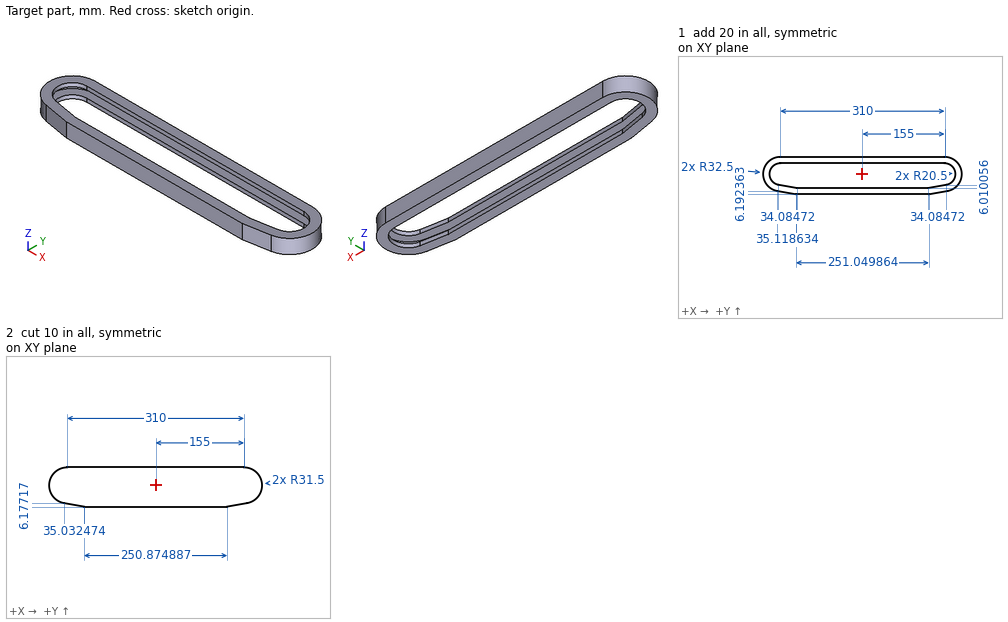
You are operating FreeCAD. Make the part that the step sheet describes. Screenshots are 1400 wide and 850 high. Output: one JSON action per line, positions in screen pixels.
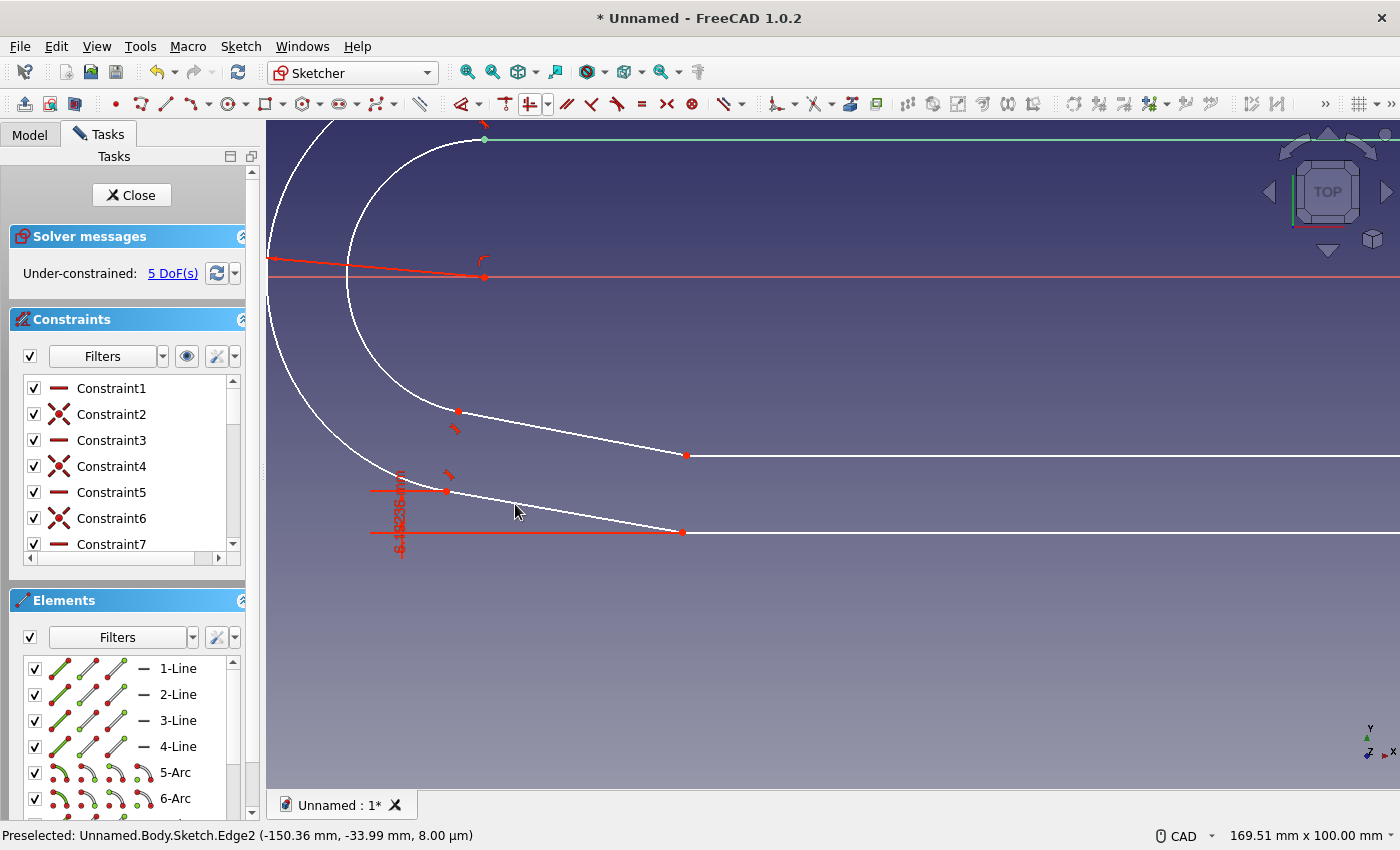
{"action": "scroll", "coordinate": [517, 506], "scroll_direction": "down", "scroll_amount": 7}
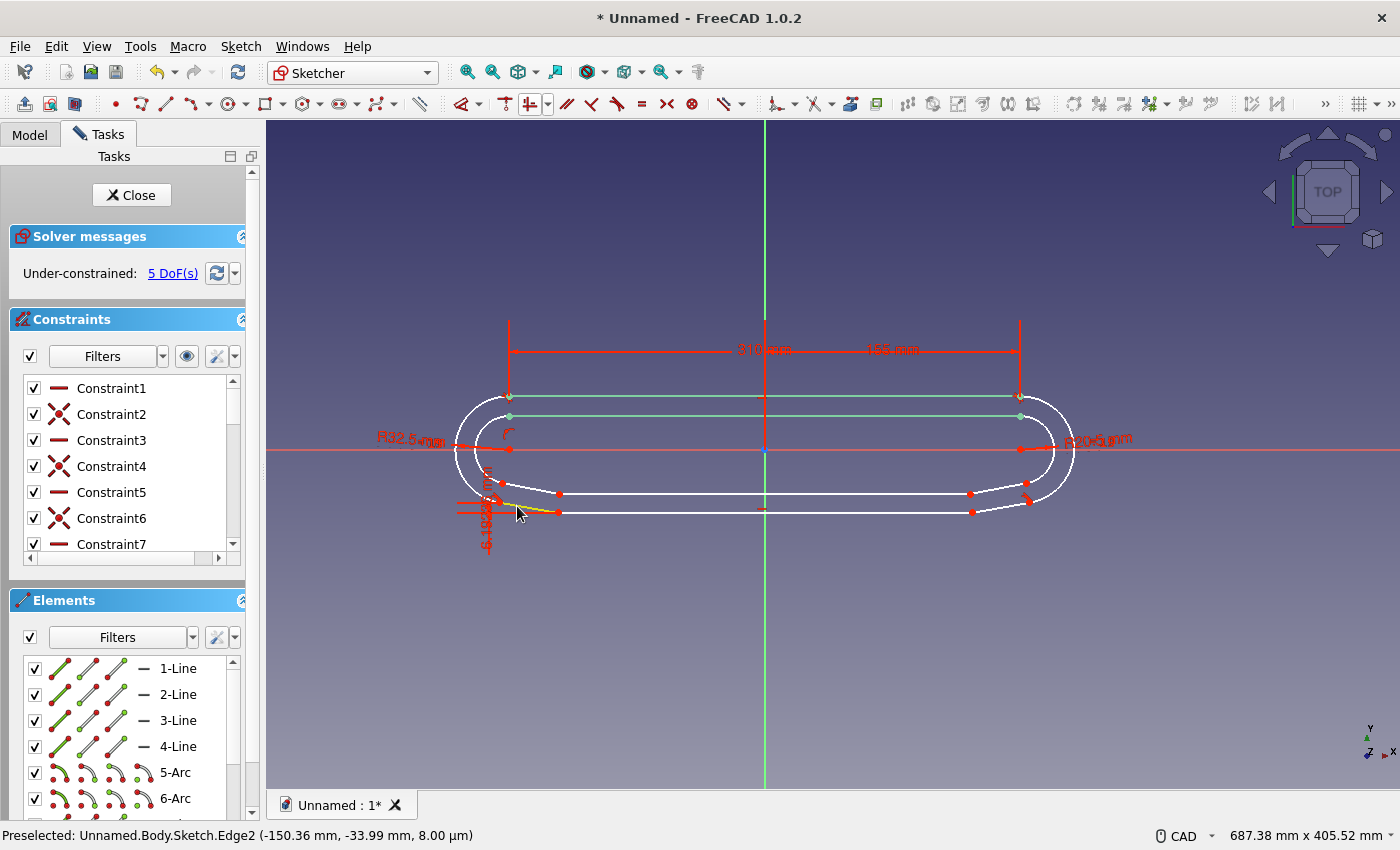
{"action": "left_click", "coordinate": [1010, 486]}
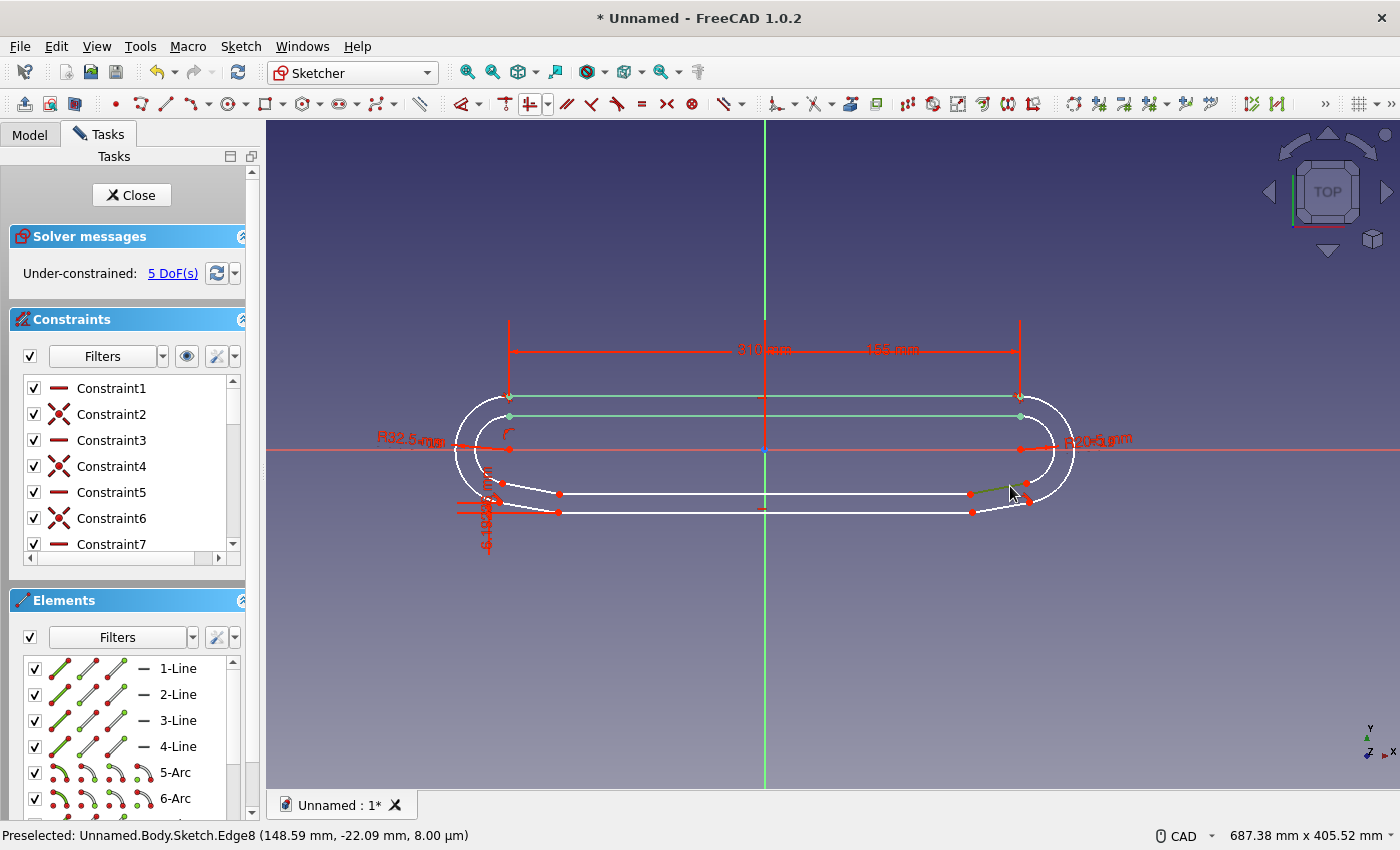
{"action": "key", "text": "l"}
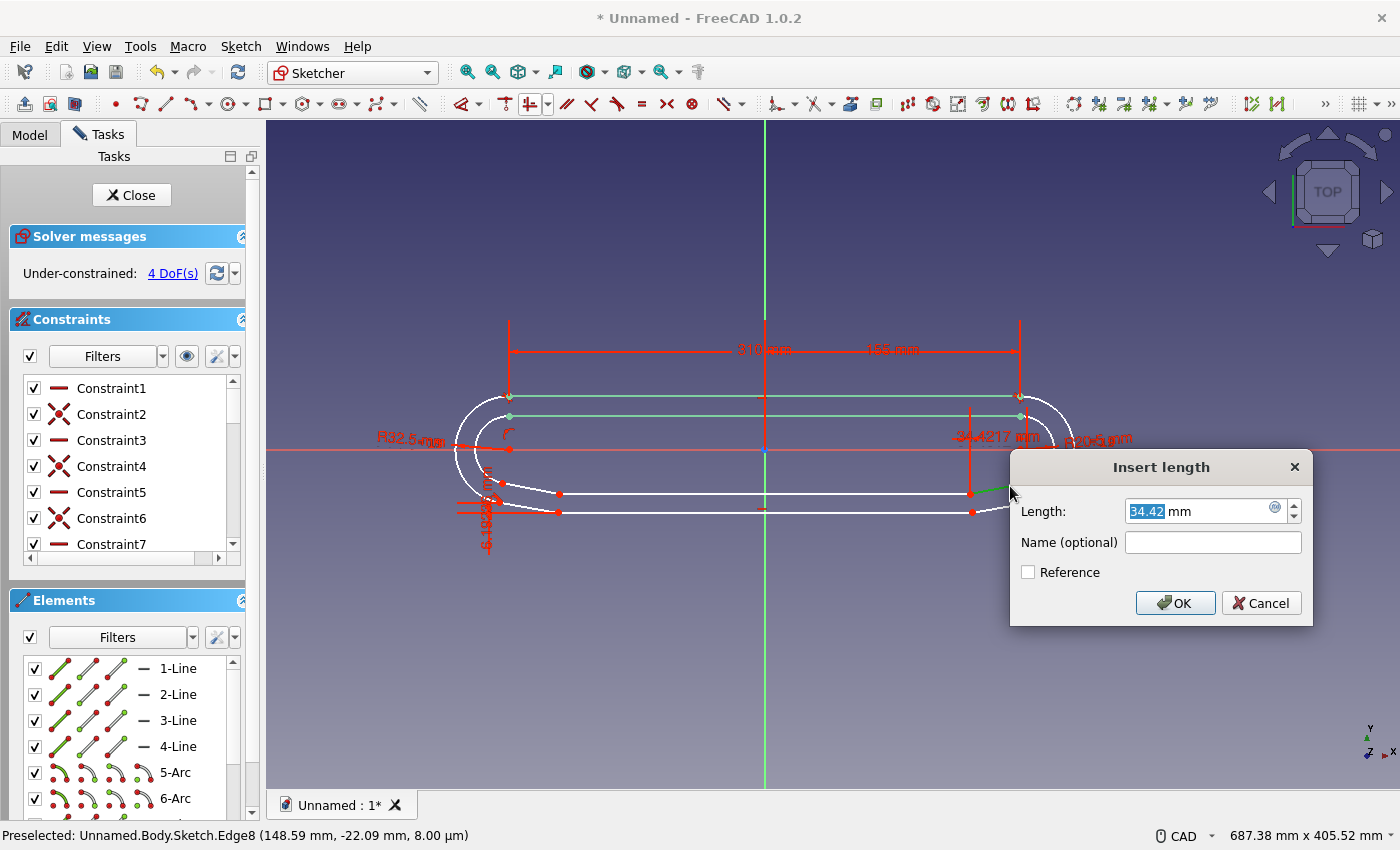
{"action": "type", "text": "34.08472"}
{"action": "key", "text": "Return"}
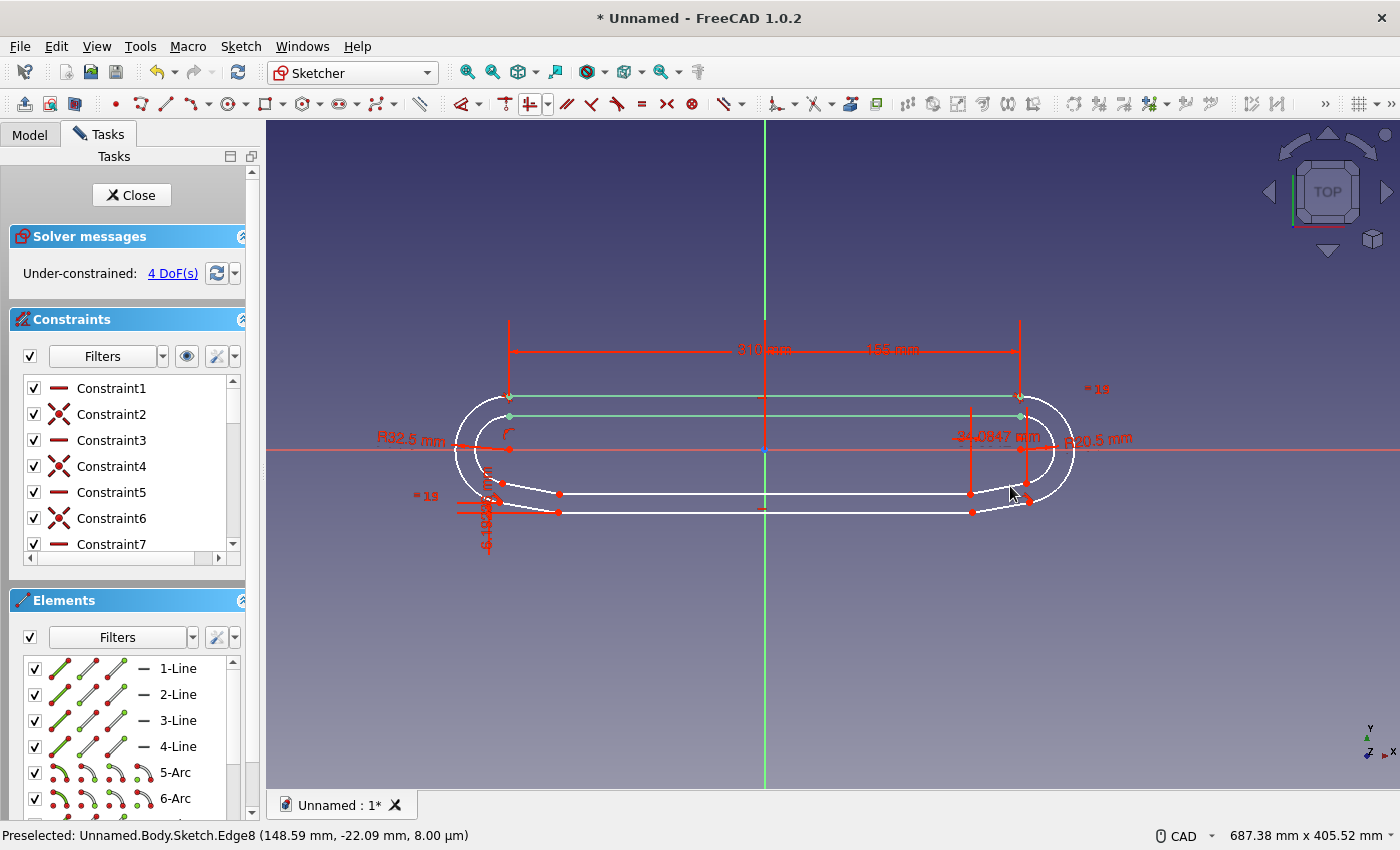
{"action": "scroll", "coordinate": [1010, 486], "scroll_direction": "up", "scroll_amount": 7}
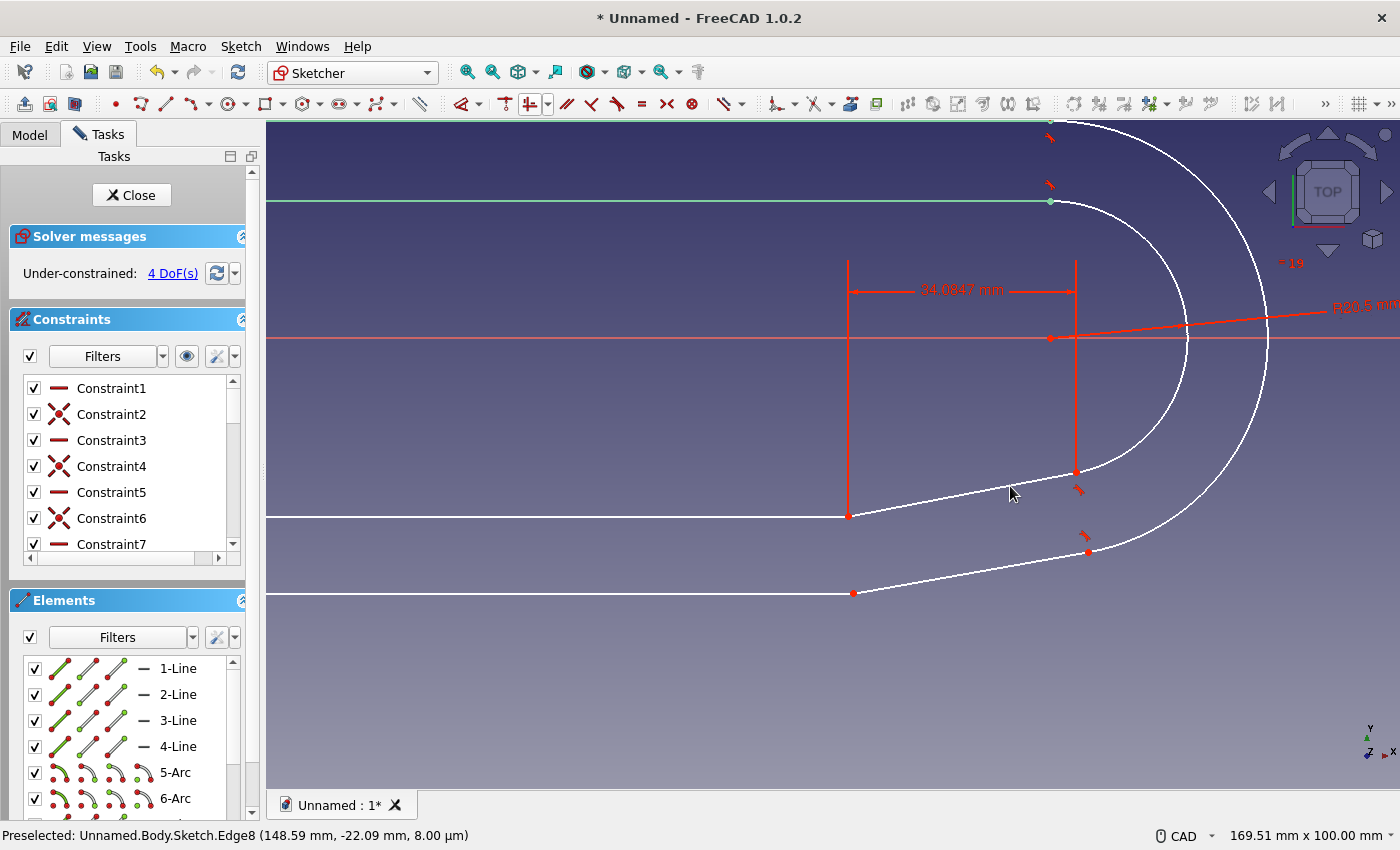
{"action": "left_click", "coordinate": [1008, 486]}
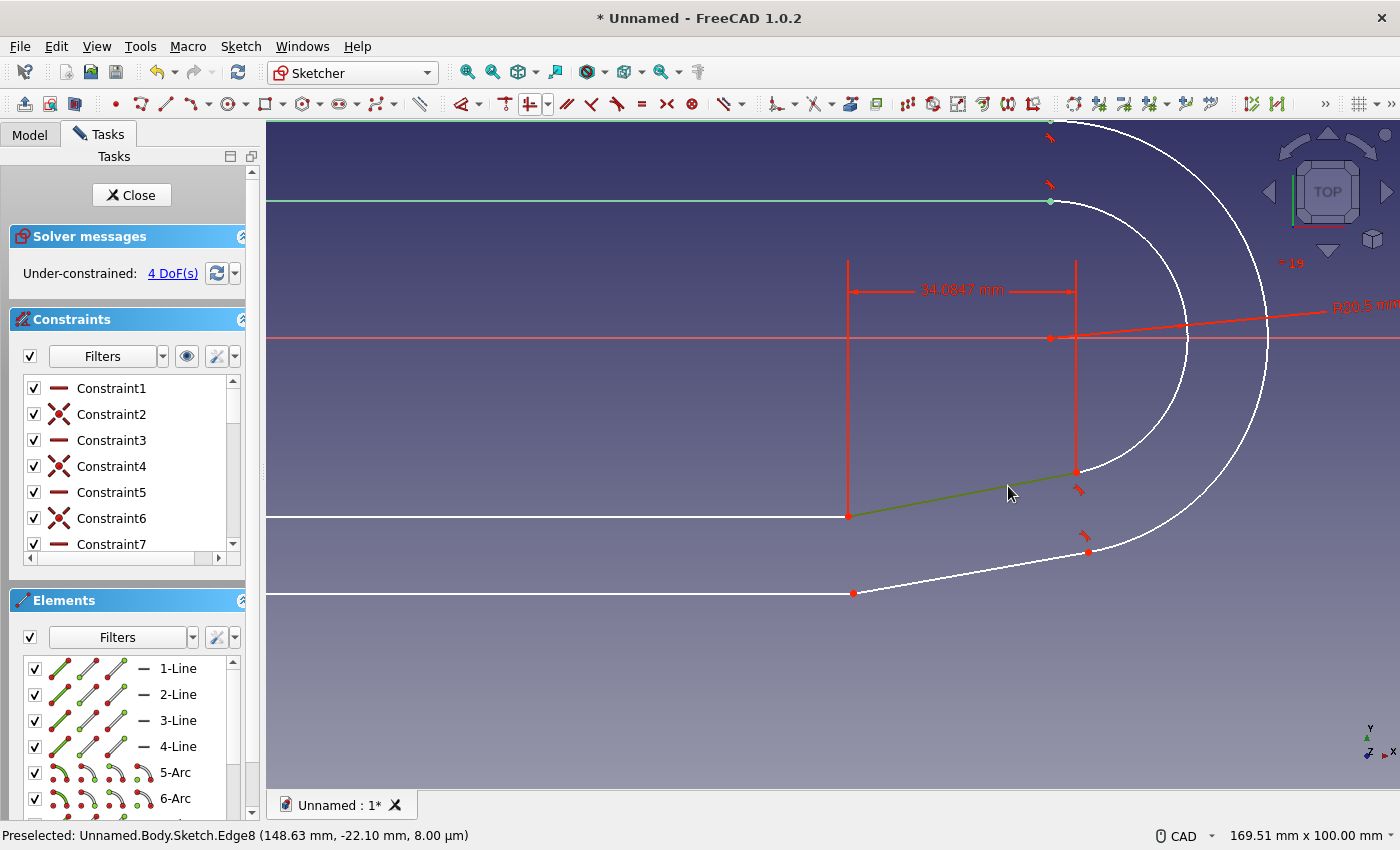
{"action": "left_click", "coordinate": [478, 104]}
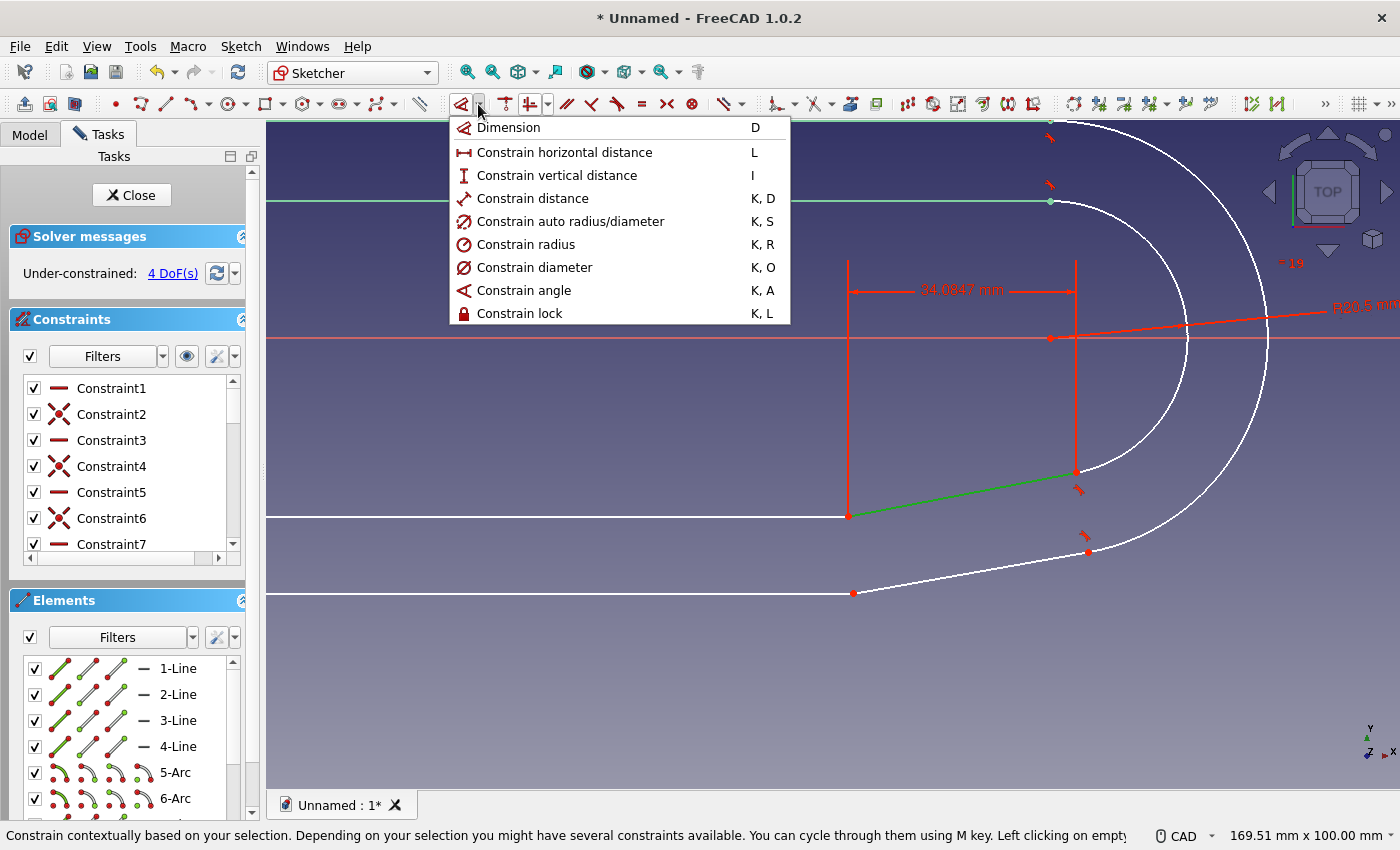
{"action": "left_click", "coordinate": [620, 176]}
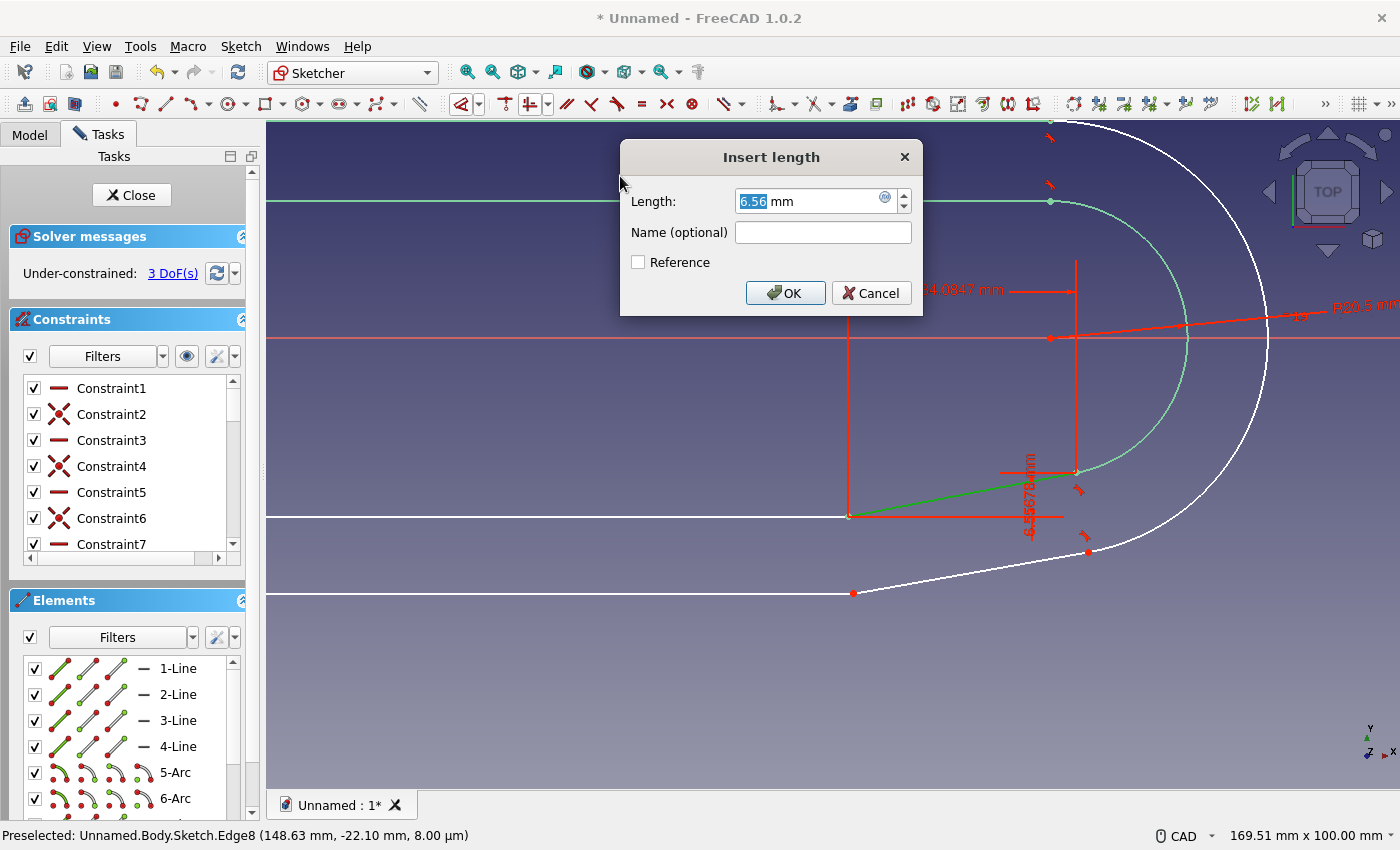
{"action": "type", "text": "6.010056"}
{"action": "key", "text": "Return"}